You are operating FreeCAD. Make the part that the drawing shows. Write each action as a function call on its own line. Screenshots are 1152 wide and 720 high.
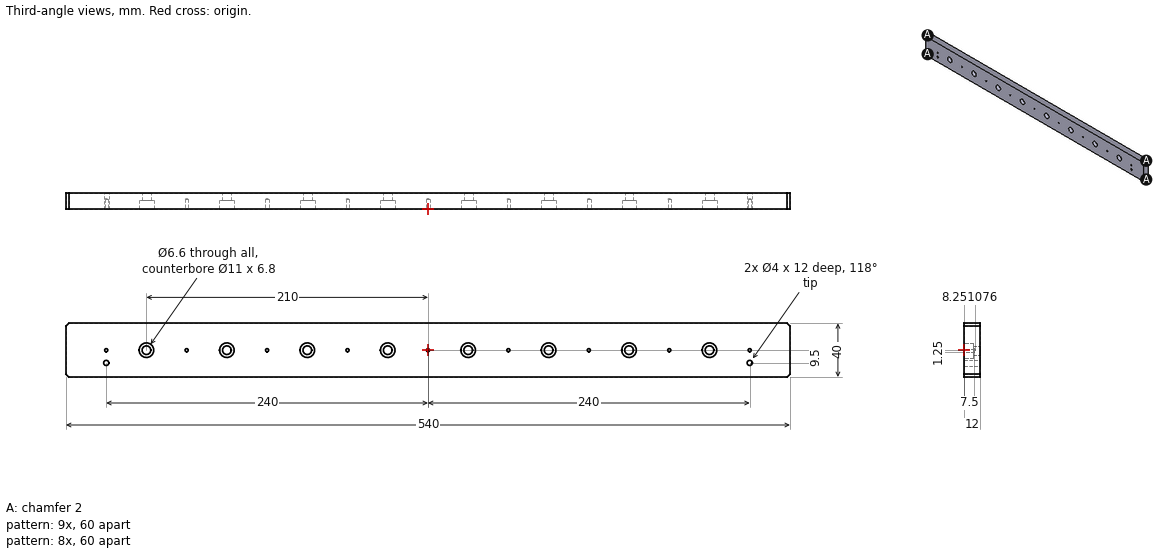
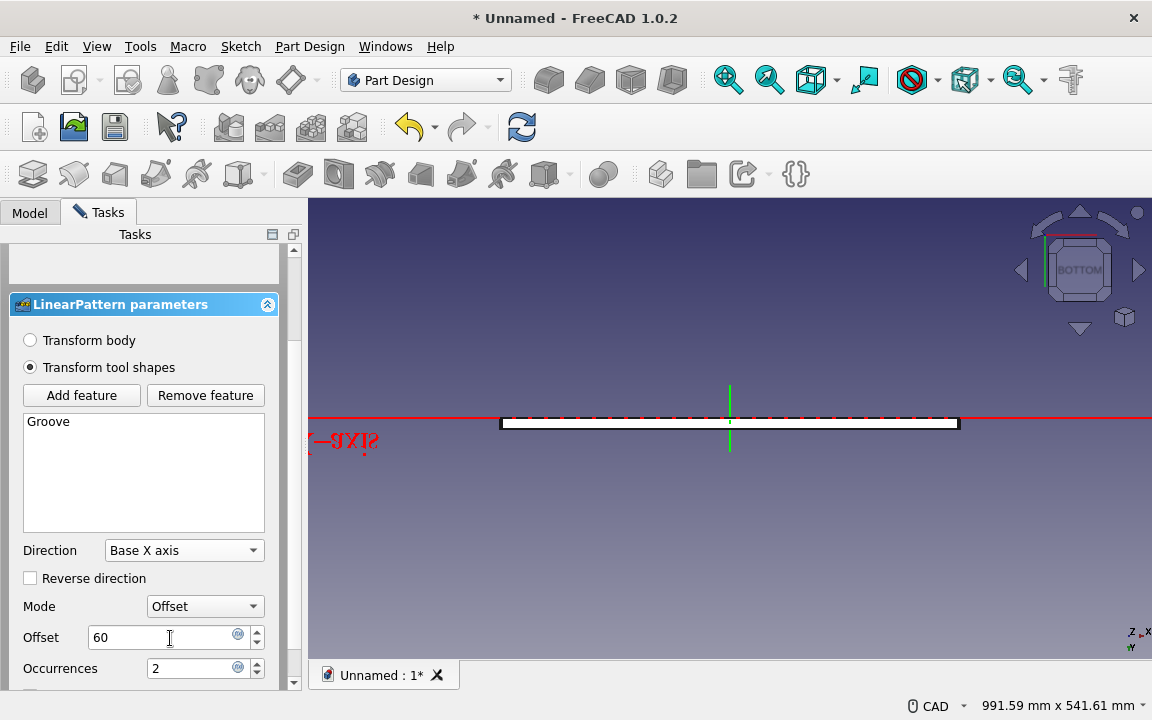
triple_click(199, 668)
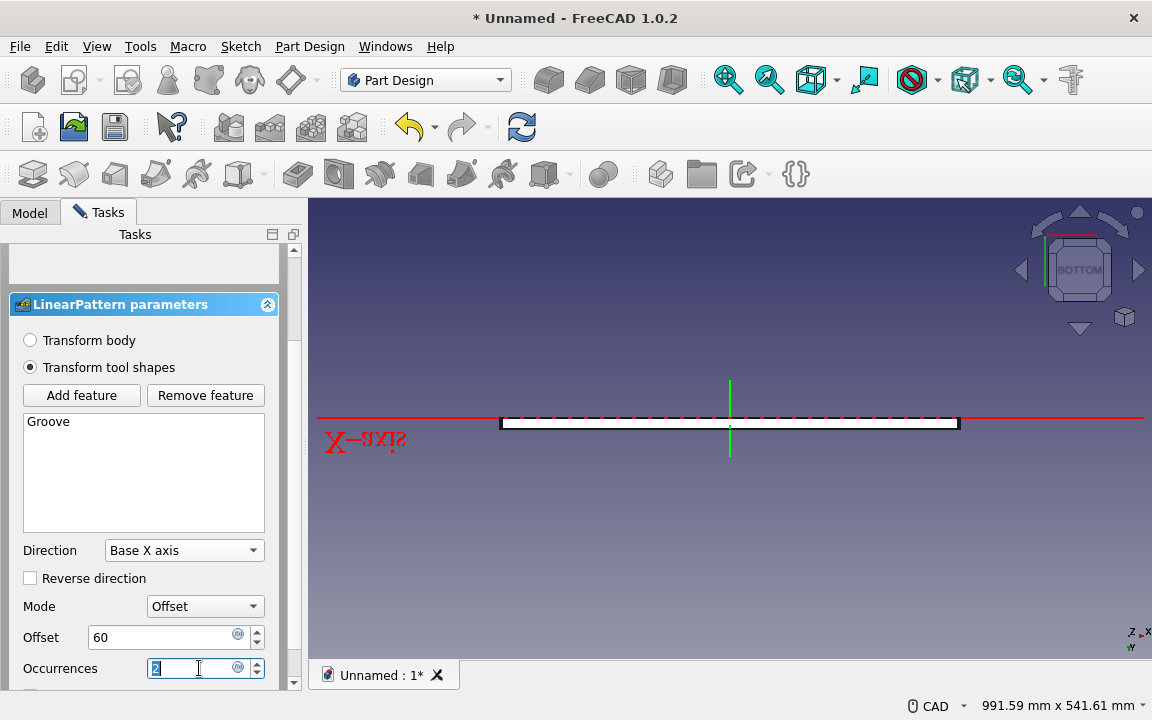
text(9)
key(Tab)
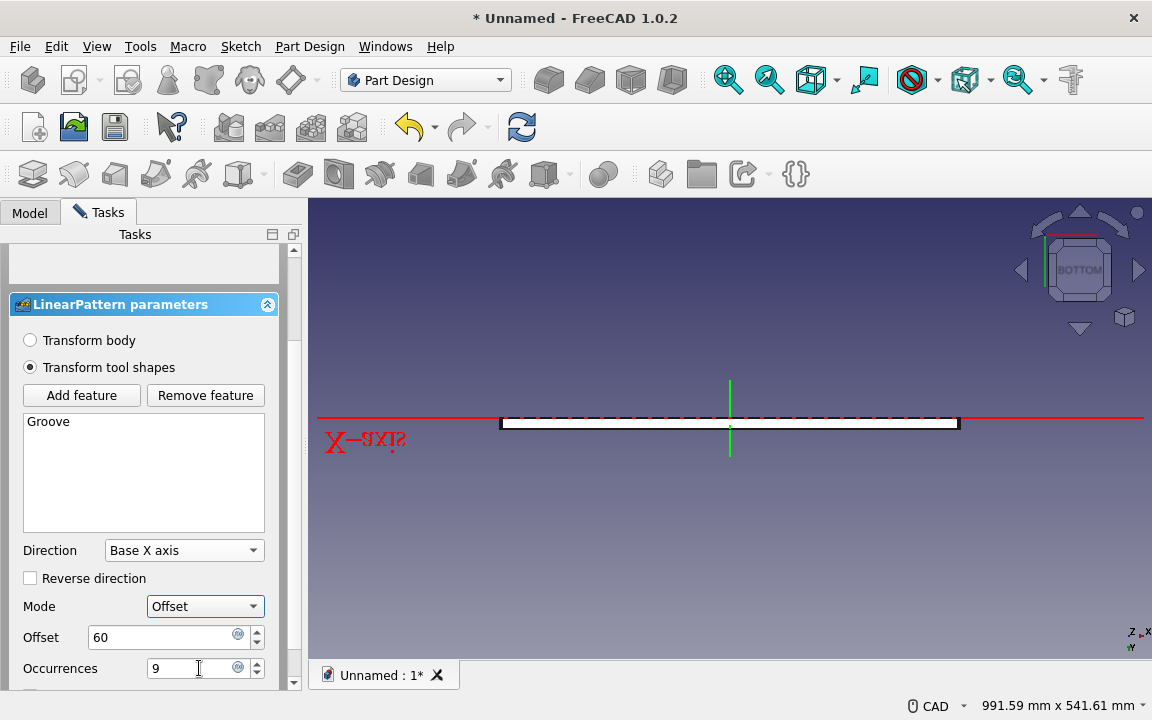
click(31, 578)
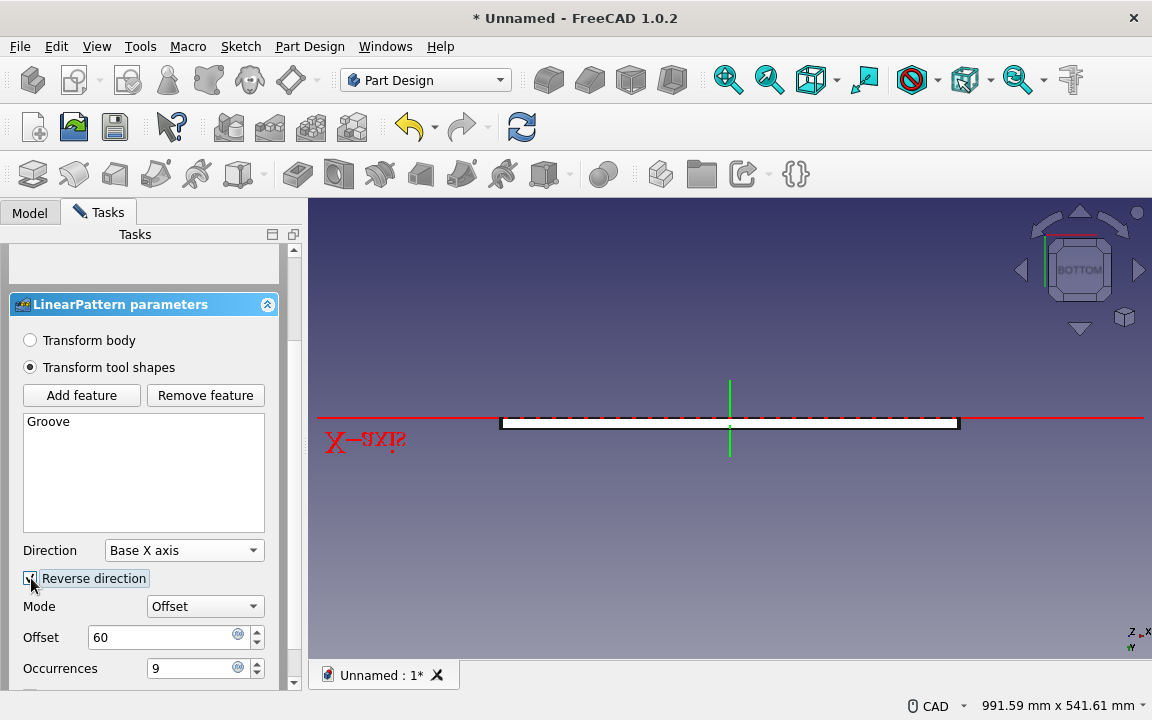
scroll(294, 467, up, 3)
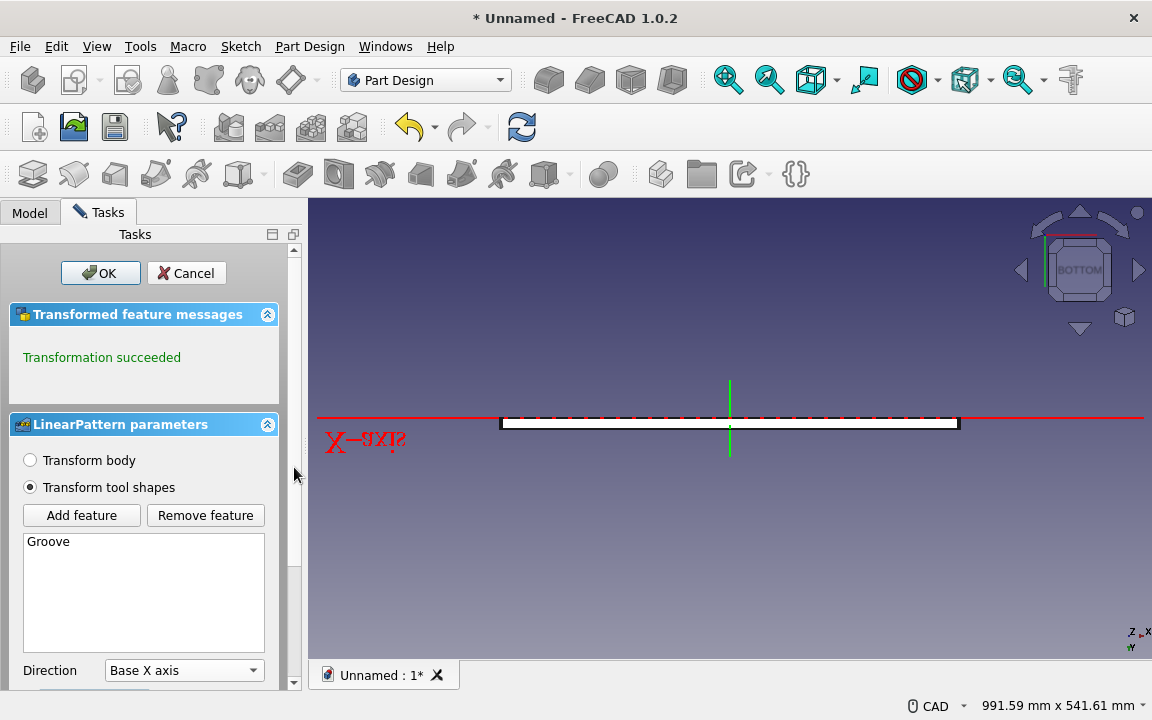
click(101, 273)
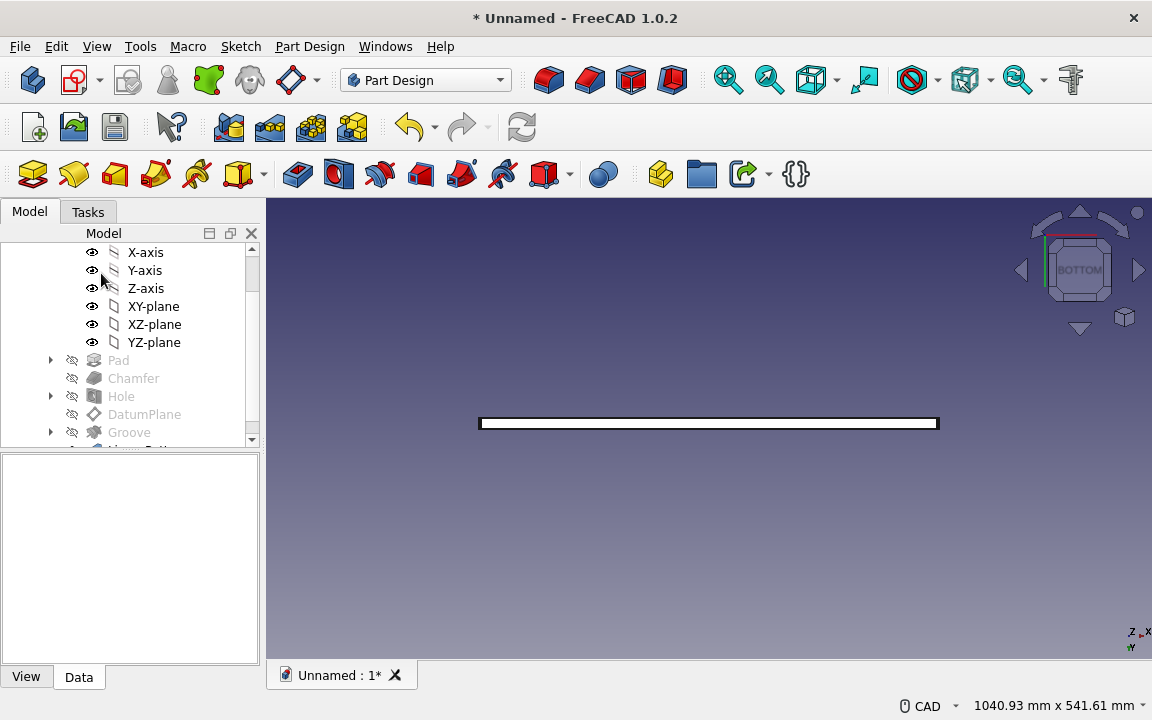
click(74, 80)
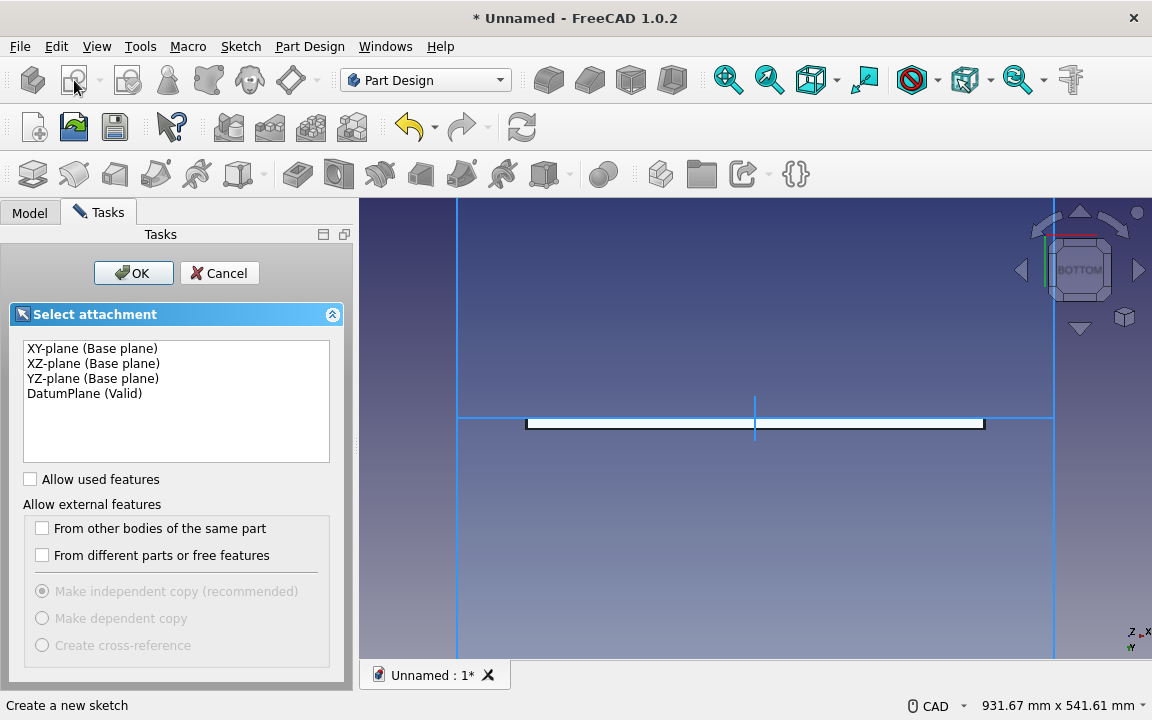
click(84, 364)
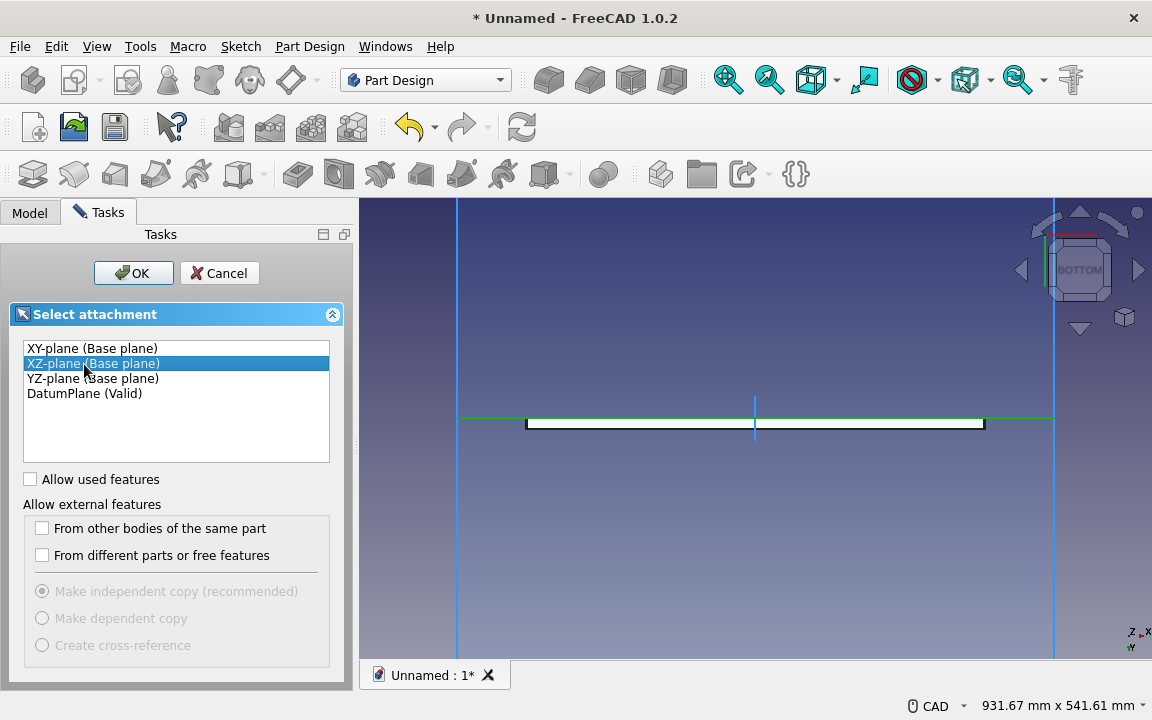
click(134, 273)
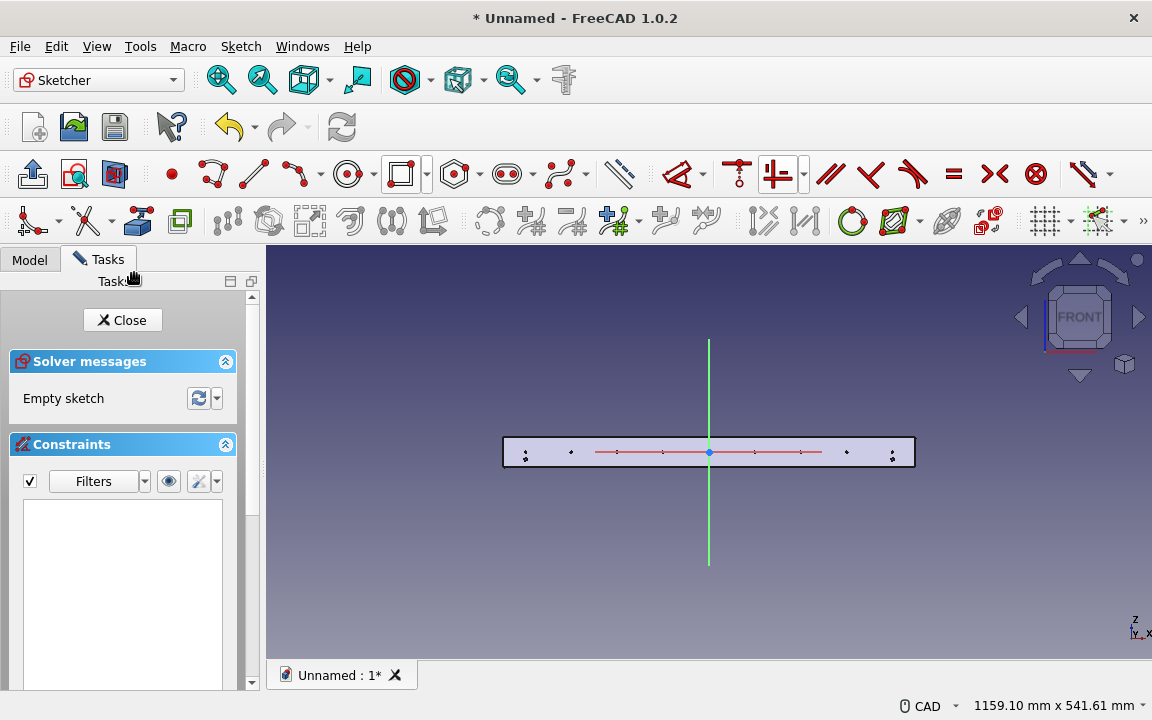
scroll(544, 452, up, 15)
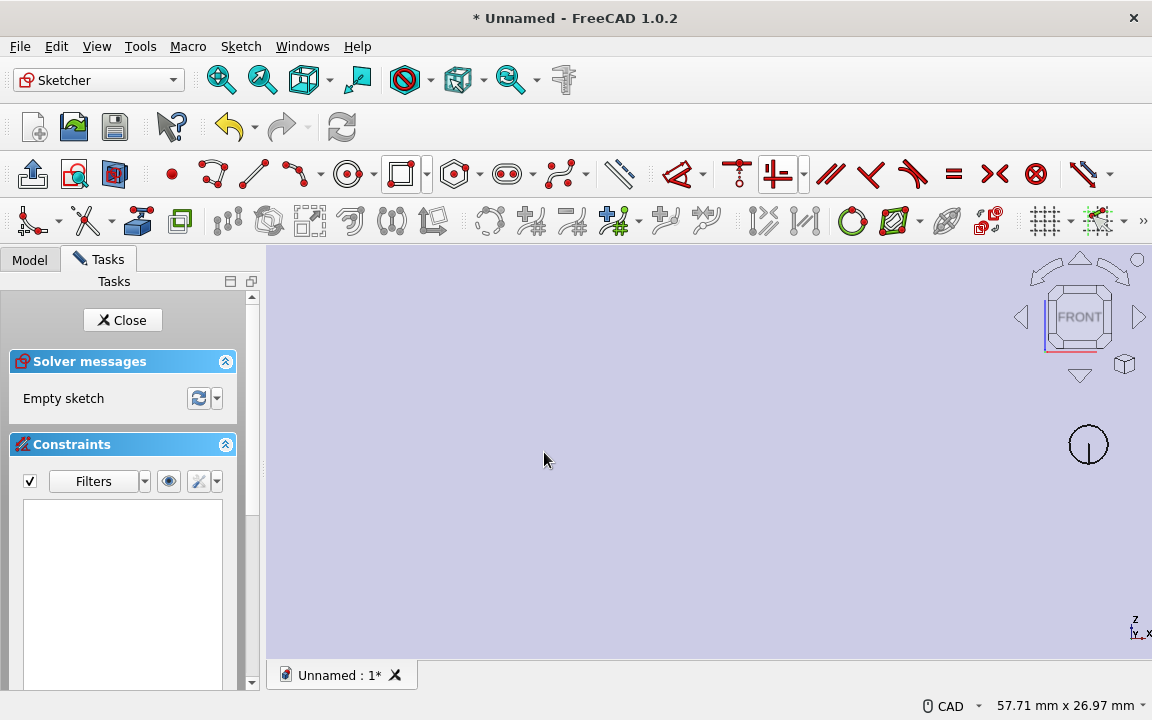
scroll(621, 440, up, 5)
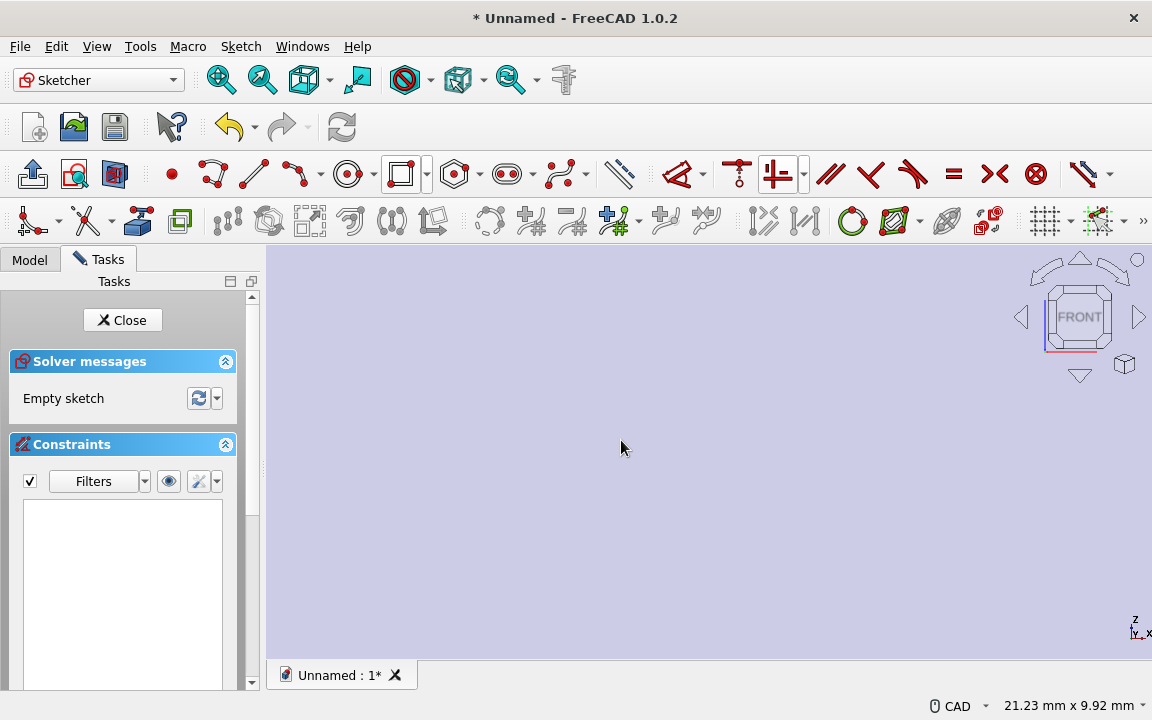
click(348, 174)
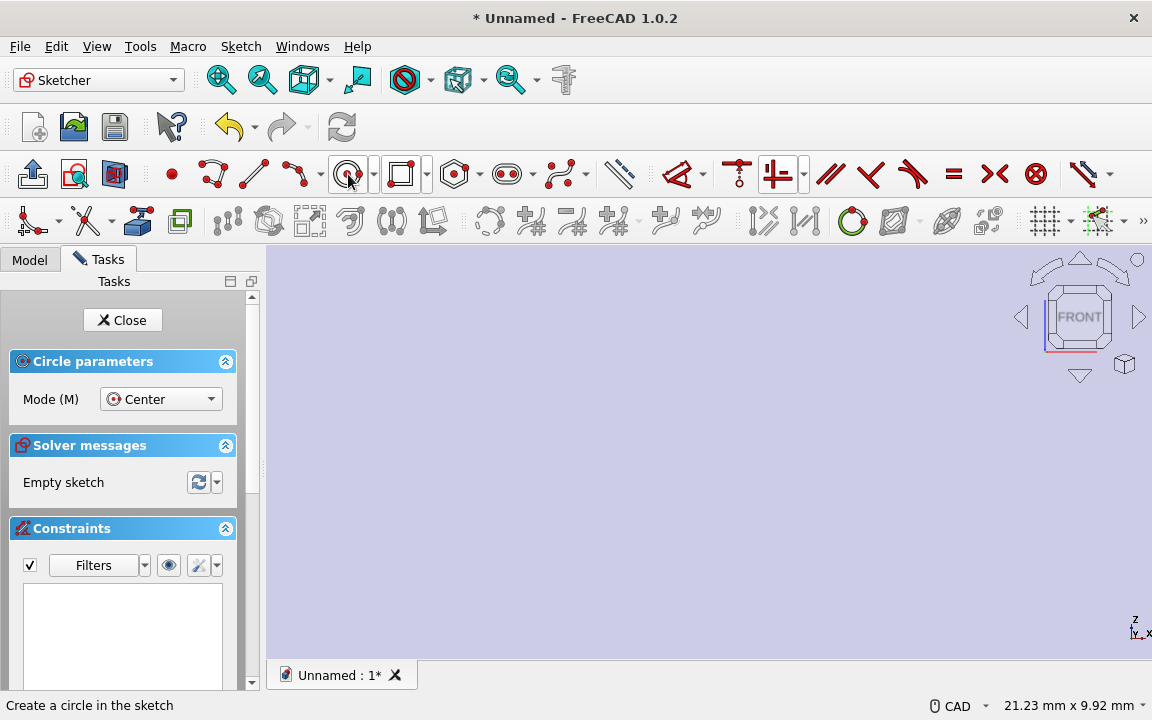
click(639, 451)
click(737, 354)
key(Escape)